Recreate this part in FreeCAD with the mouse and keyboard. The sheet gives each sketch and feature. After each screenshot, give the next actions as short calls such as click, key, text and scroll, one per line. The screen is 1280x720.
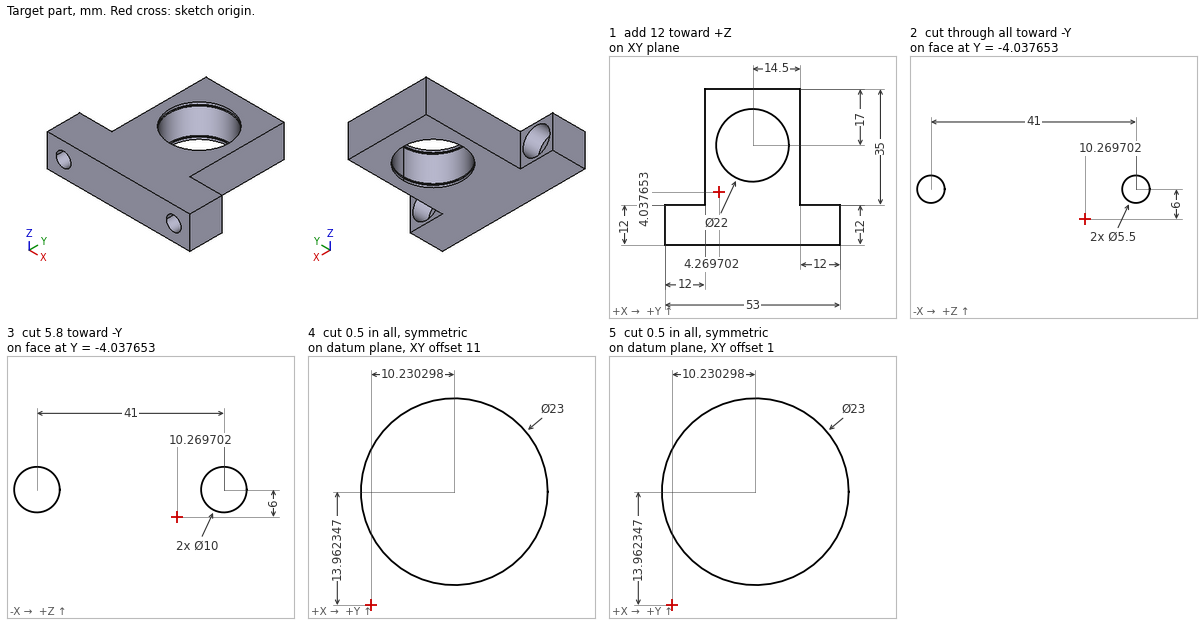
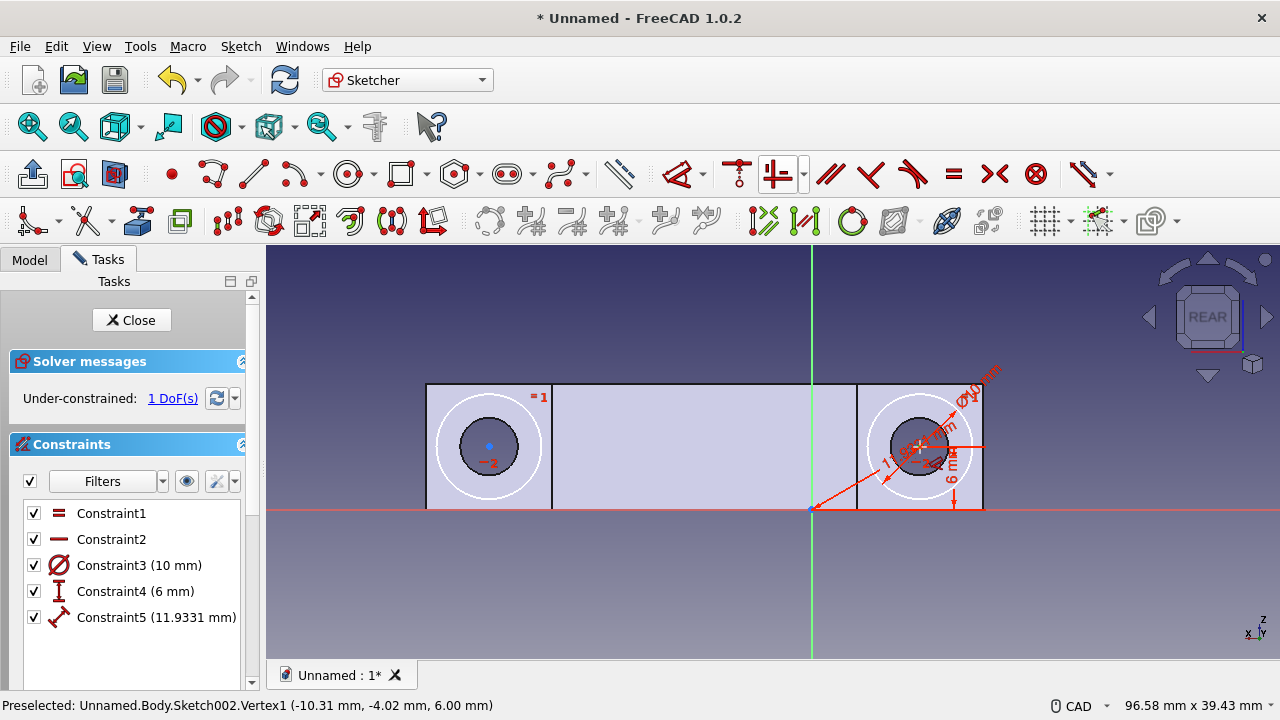
click(489, 447)
click(705, 413)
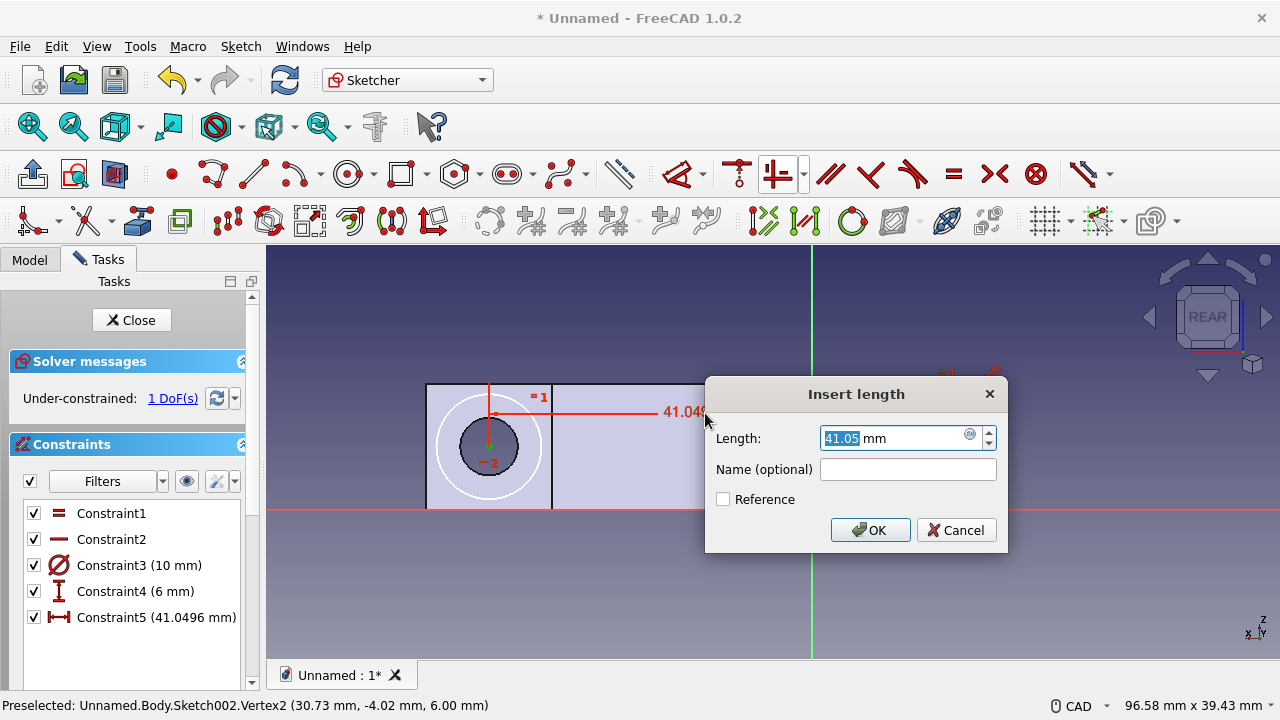
text(41)
key(Return)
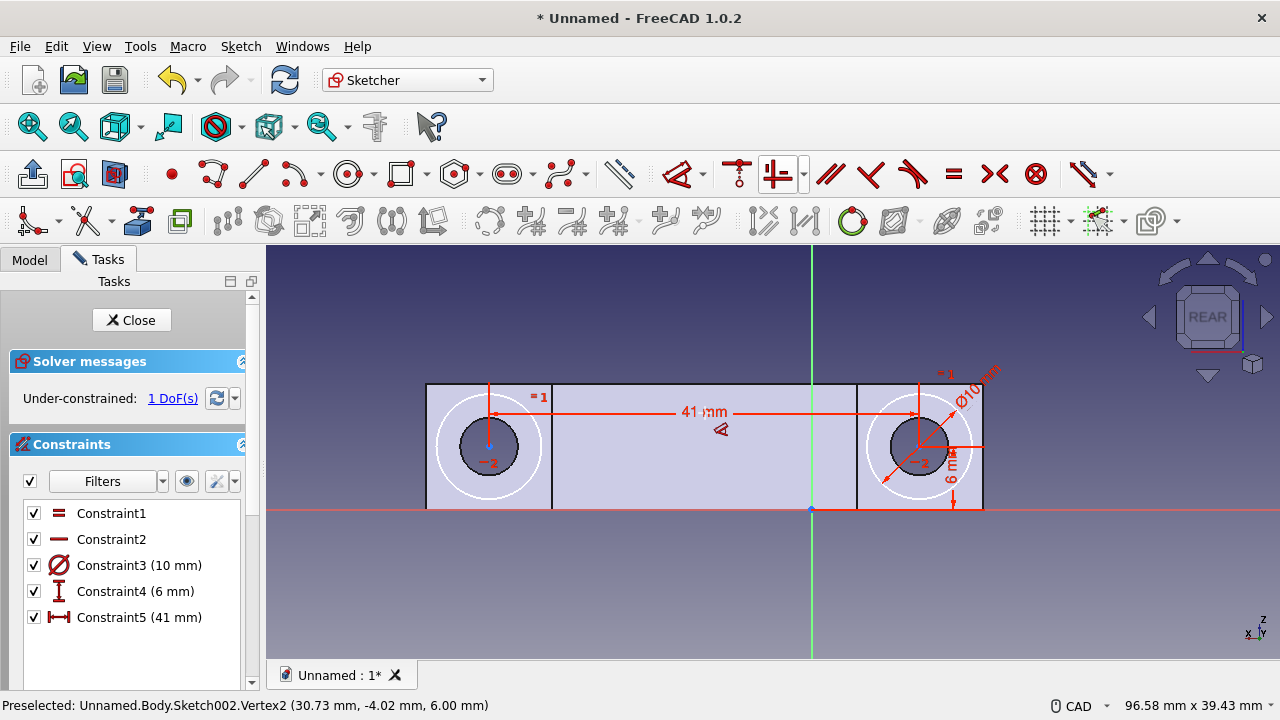
click(919, 447)
click(866, 544)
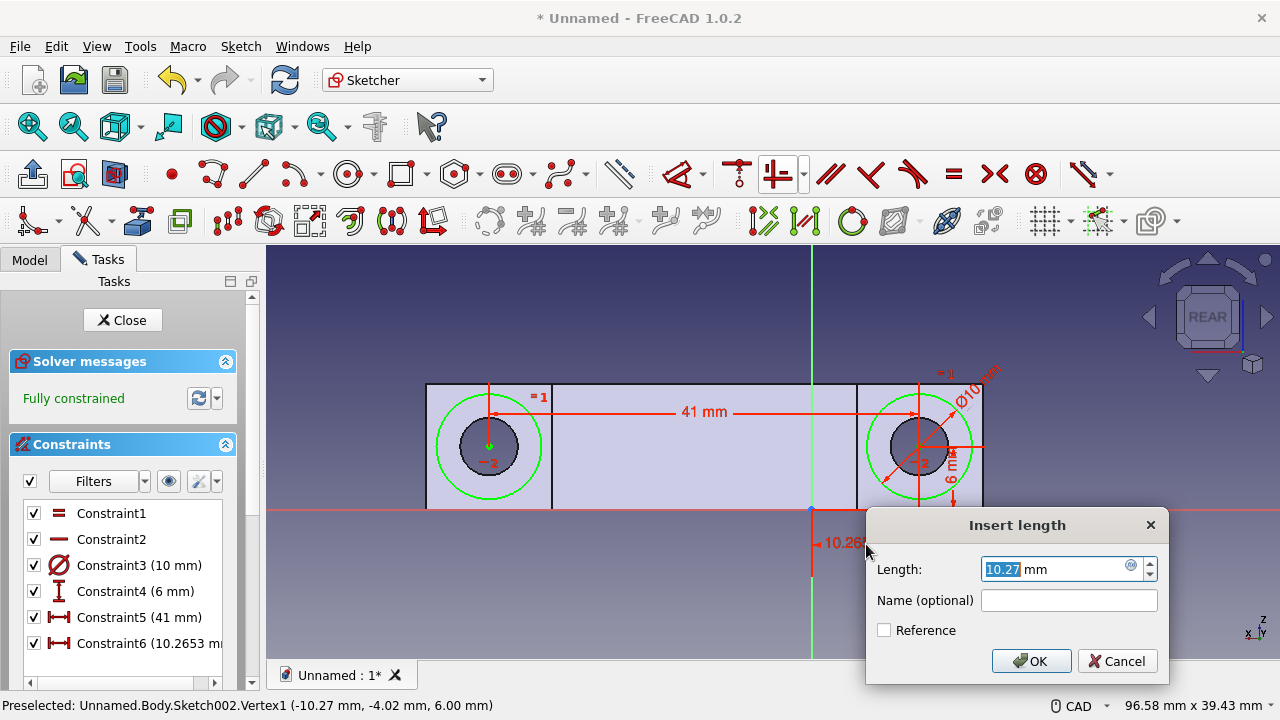
text(10.269702)
key(Return)
key(Escape)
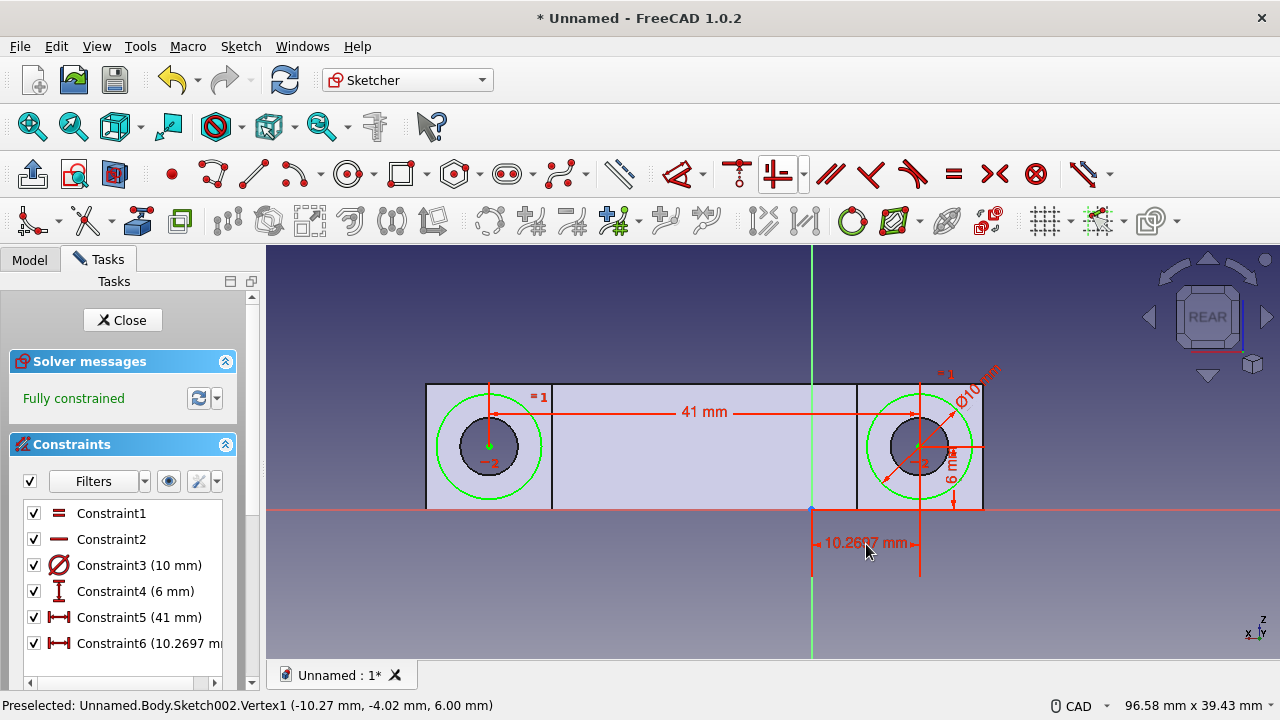
click(123, 320)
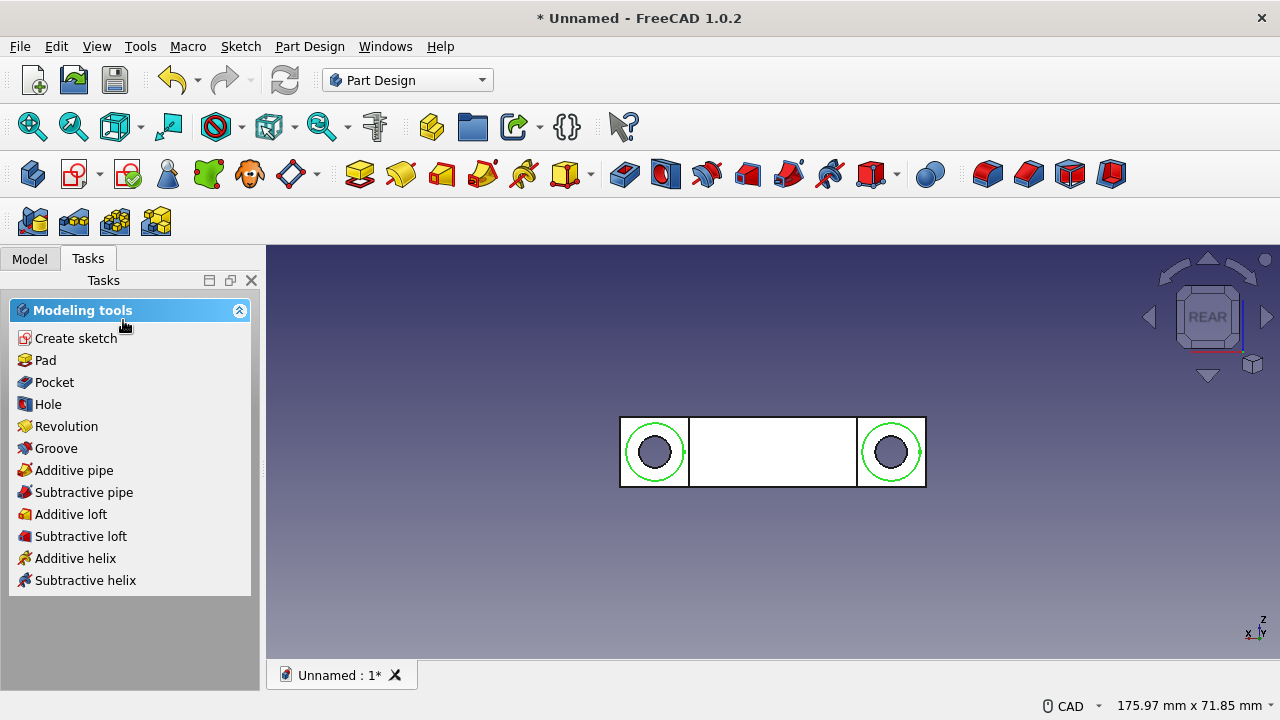
click(625, 174)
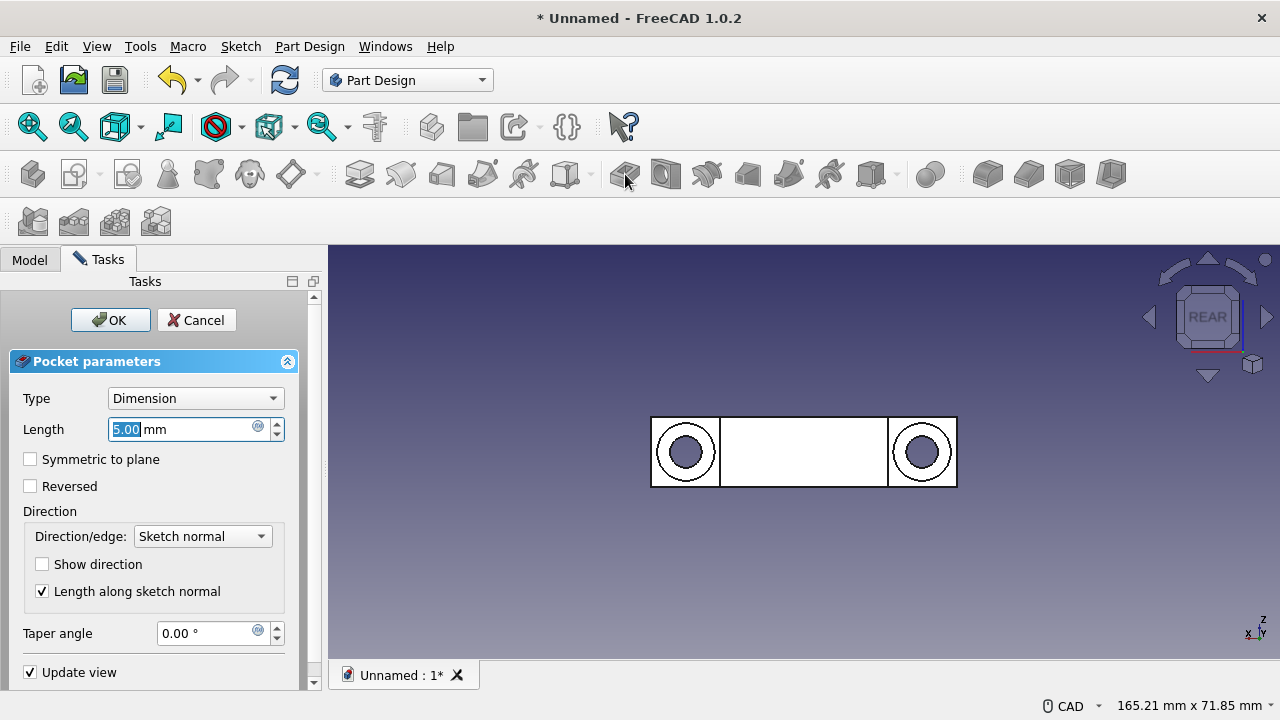
text(5.8)
key(Tab)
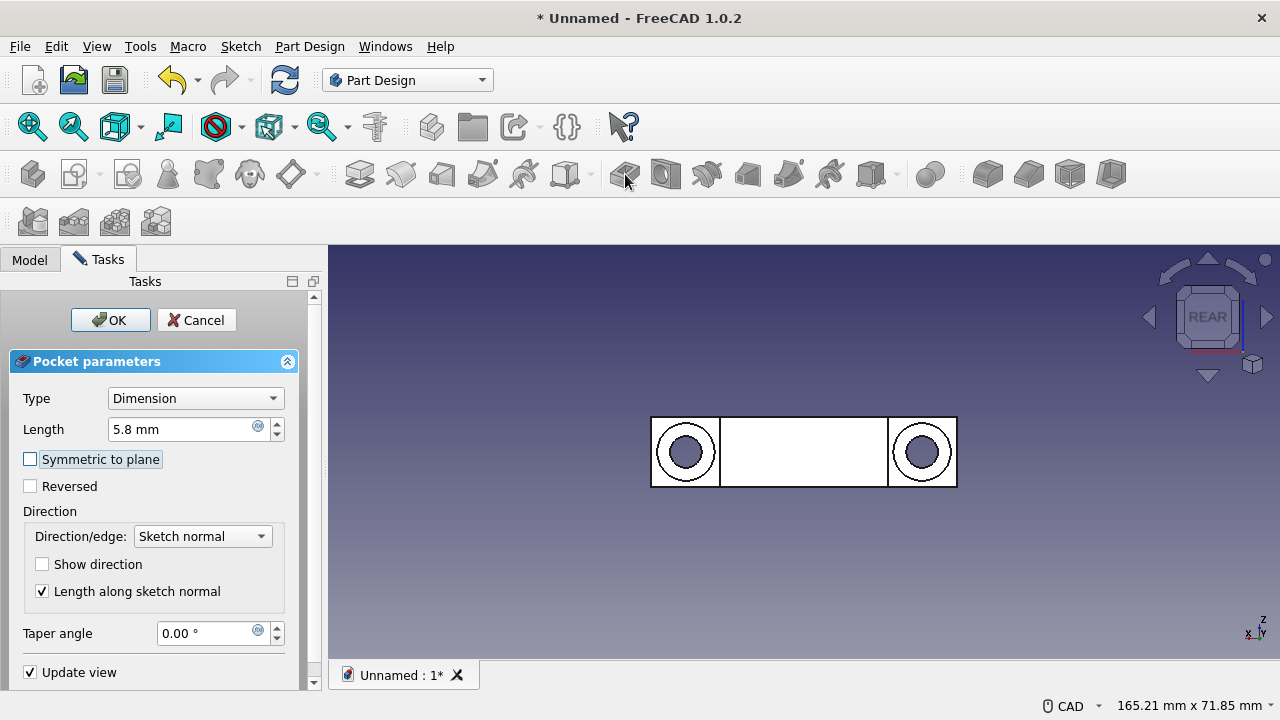
click(111, 320)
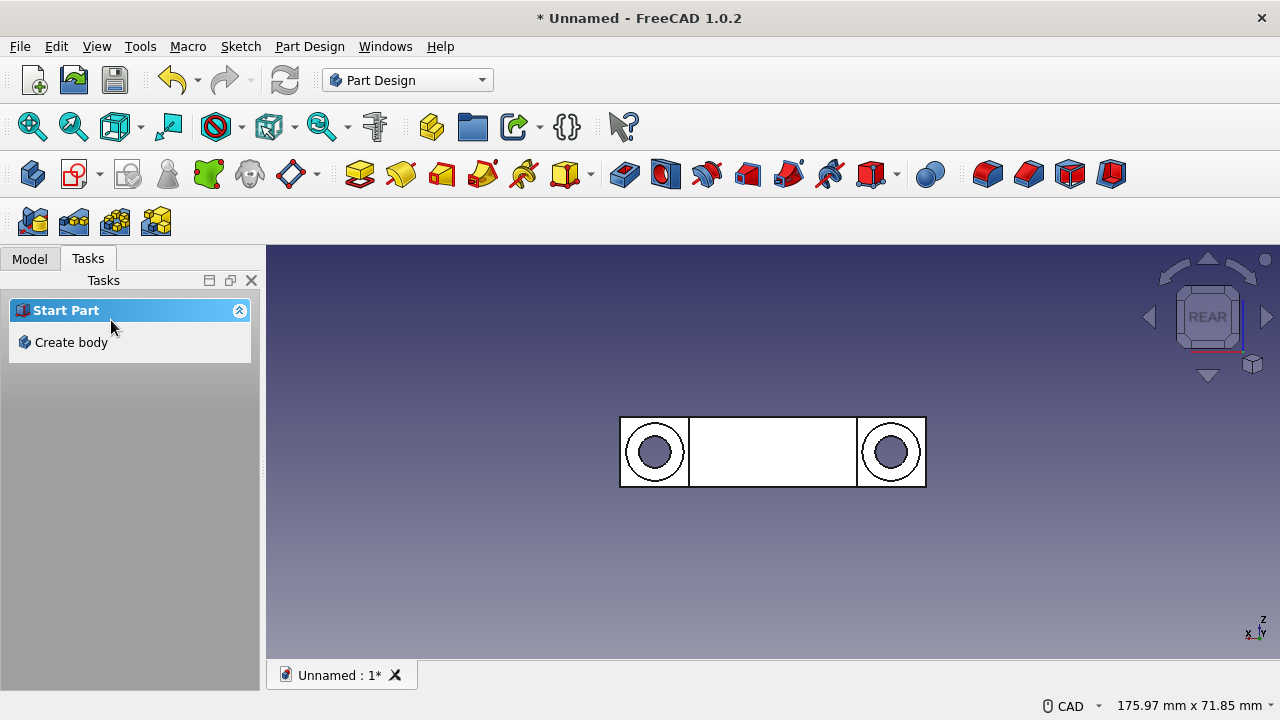
click(33, 128)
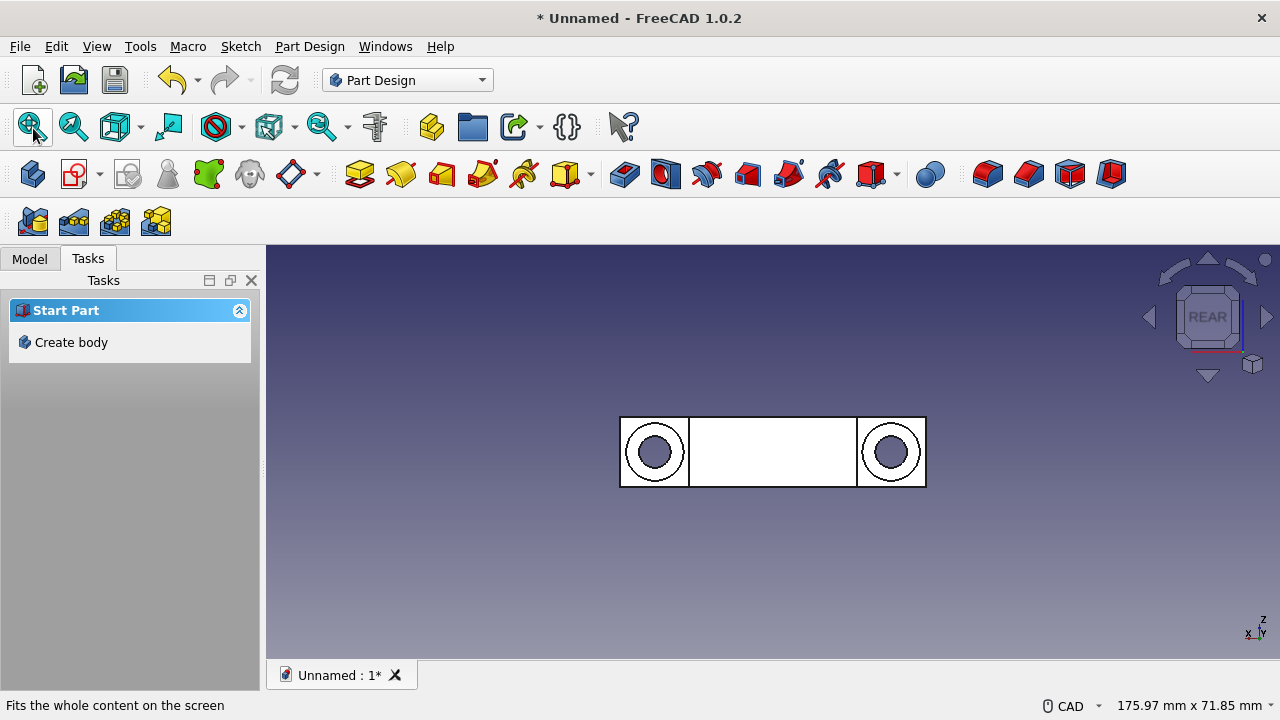
click(30, 258)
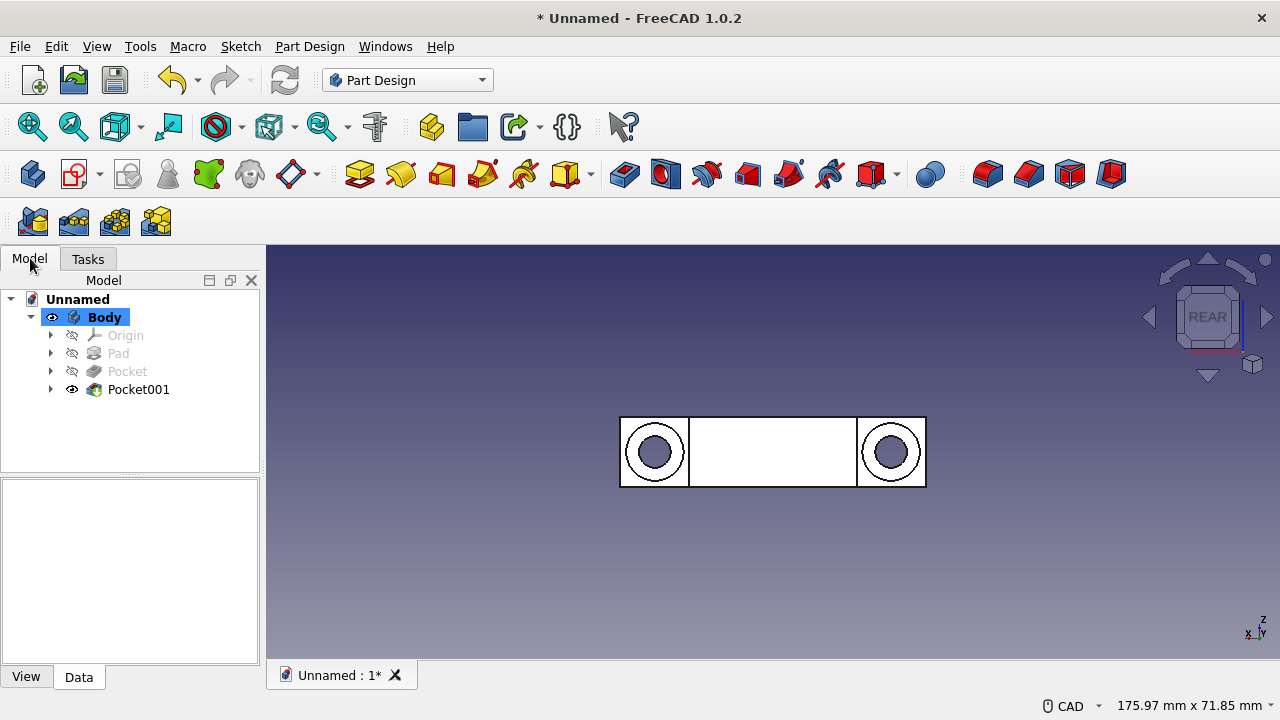
click(51, 335)